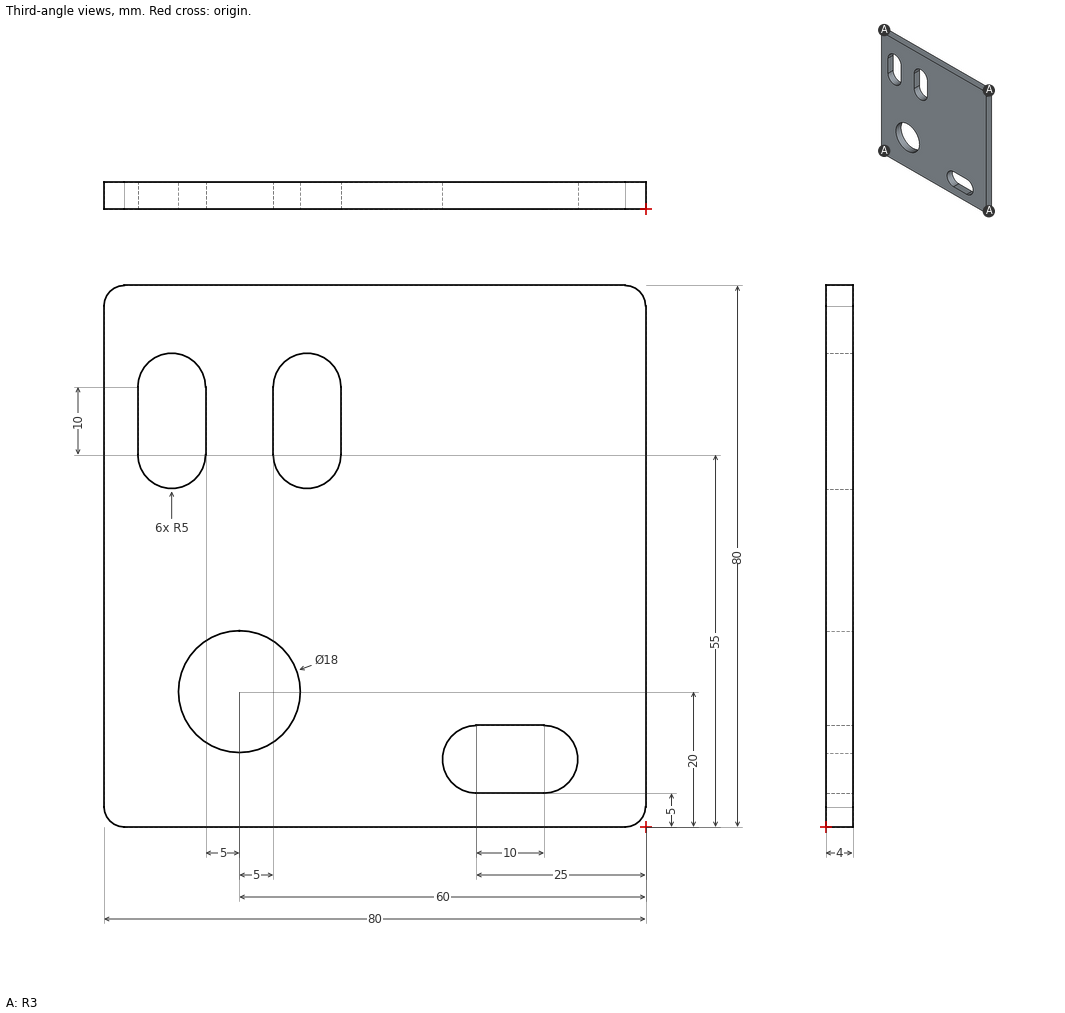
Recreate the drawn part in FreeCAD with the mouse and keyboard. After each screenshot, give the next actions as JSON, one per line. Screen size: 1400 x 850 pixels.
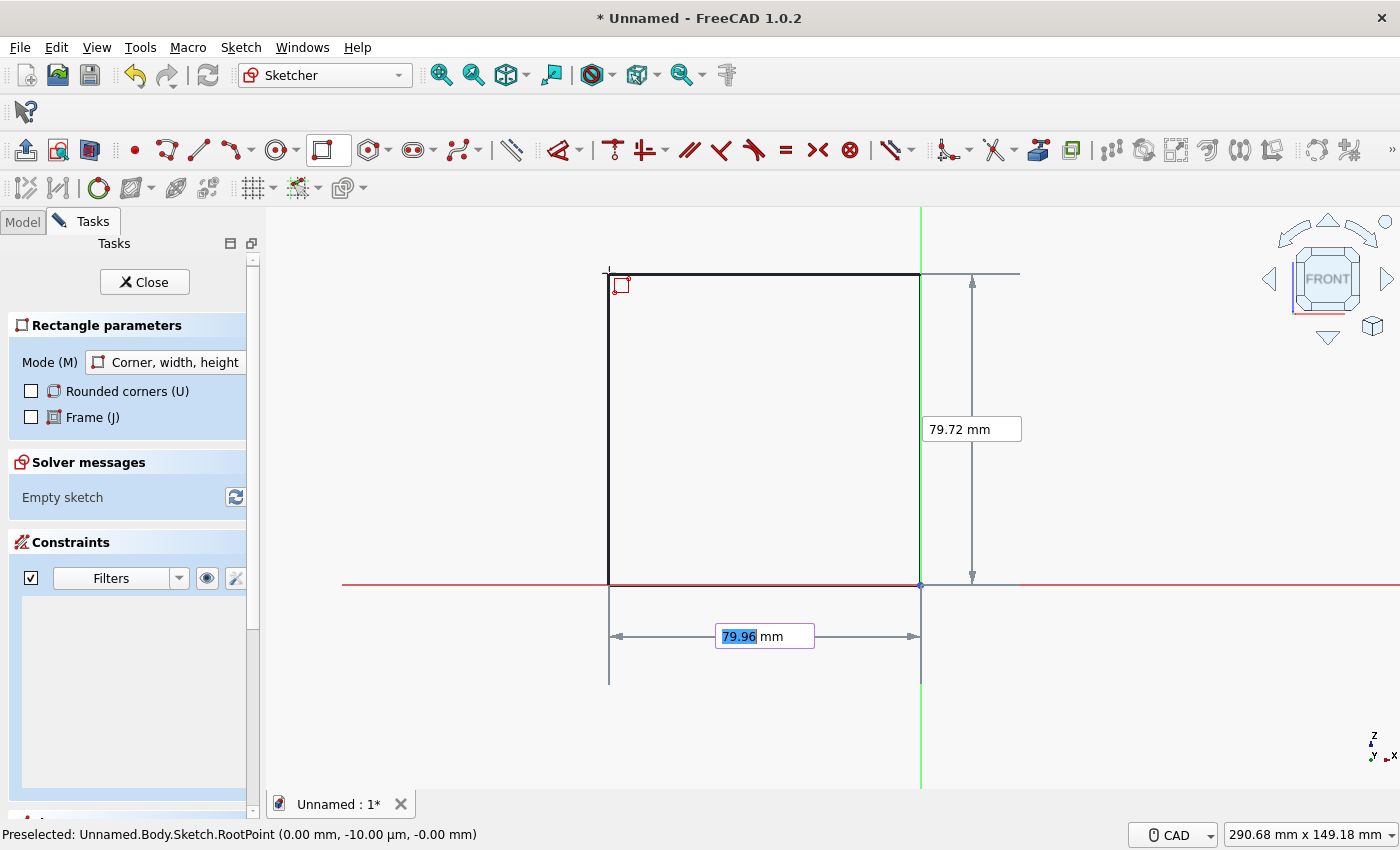
{"action": "type", "text": "80"}
{"action": "key", "text": "Tab"}
{"action": "type", "text": "80"}
{"action": "key", "text": "Return"}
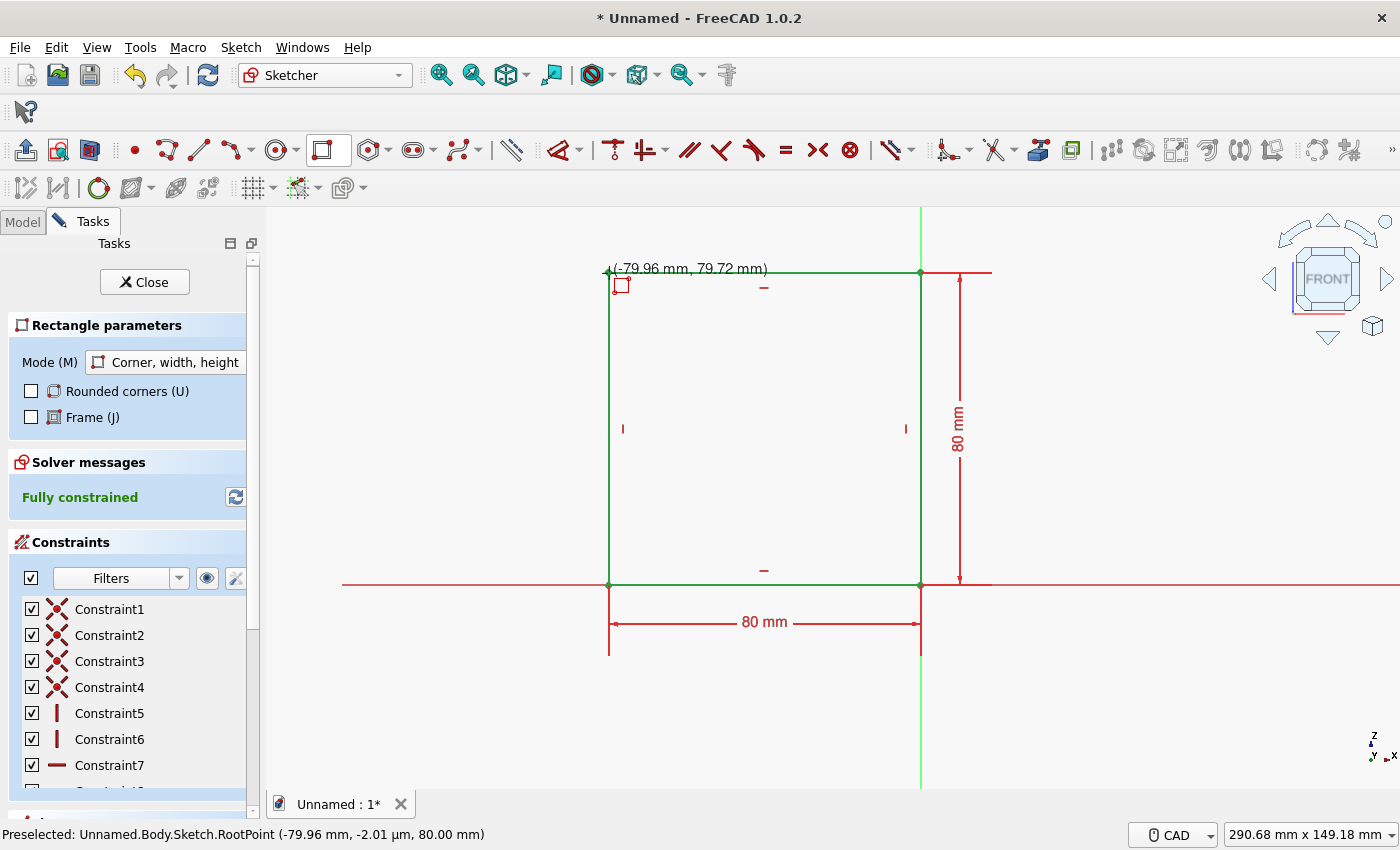
{"action": "left_click", "coordinate": [414, 150]}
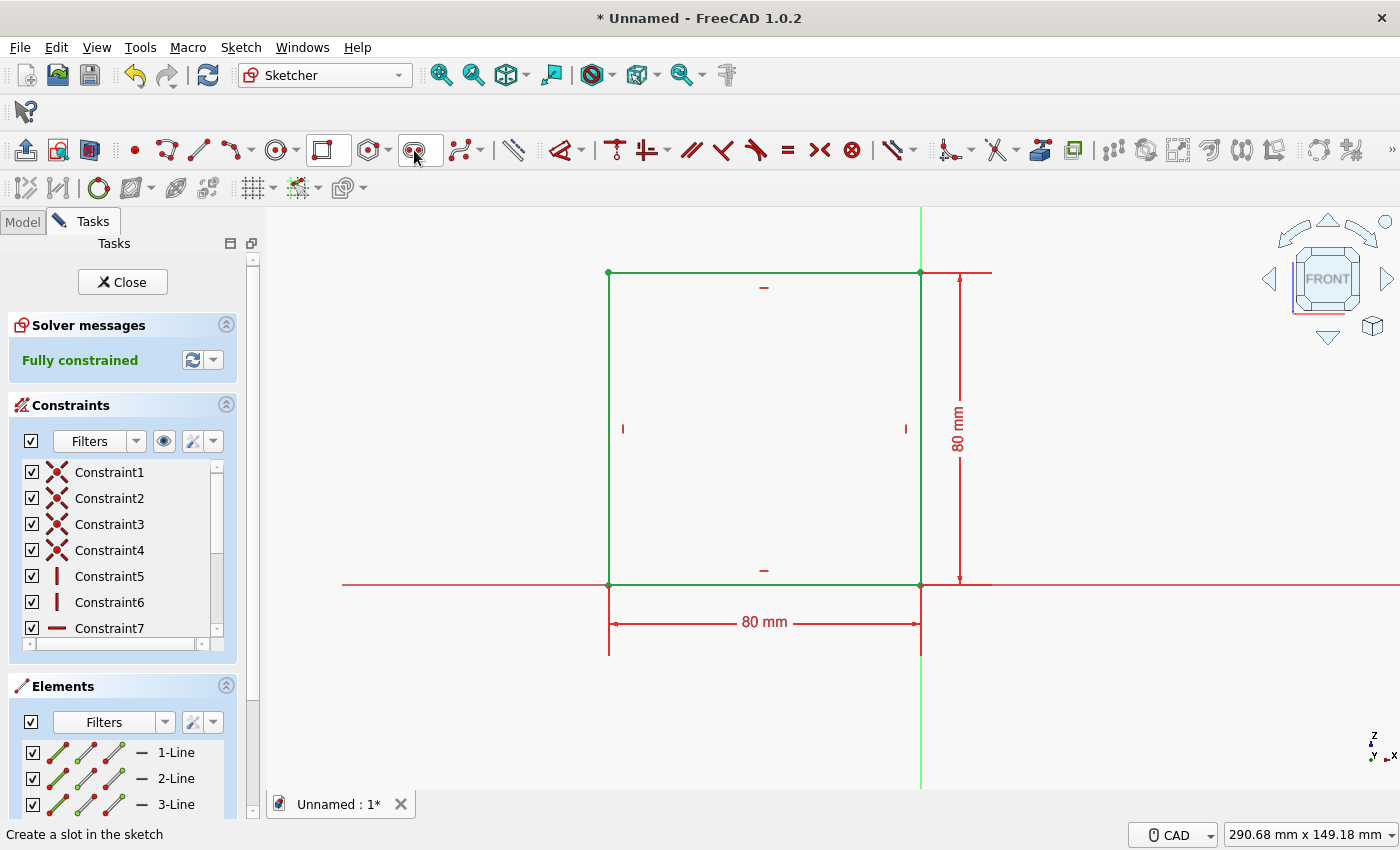
{"action": "left_click", "coordinate": [648, 370]}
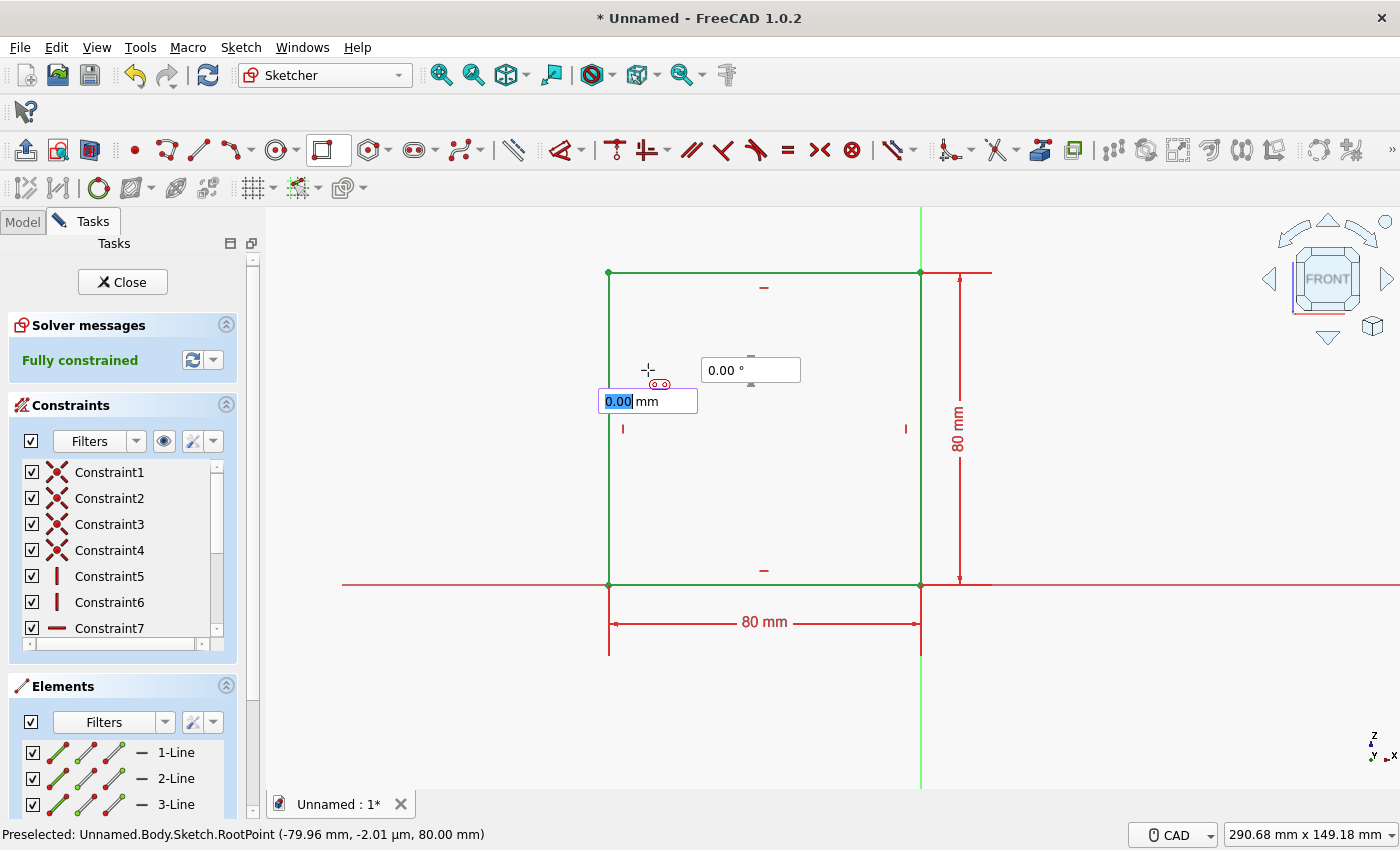
{"action": "left_click", "coordinate": [648, 331]}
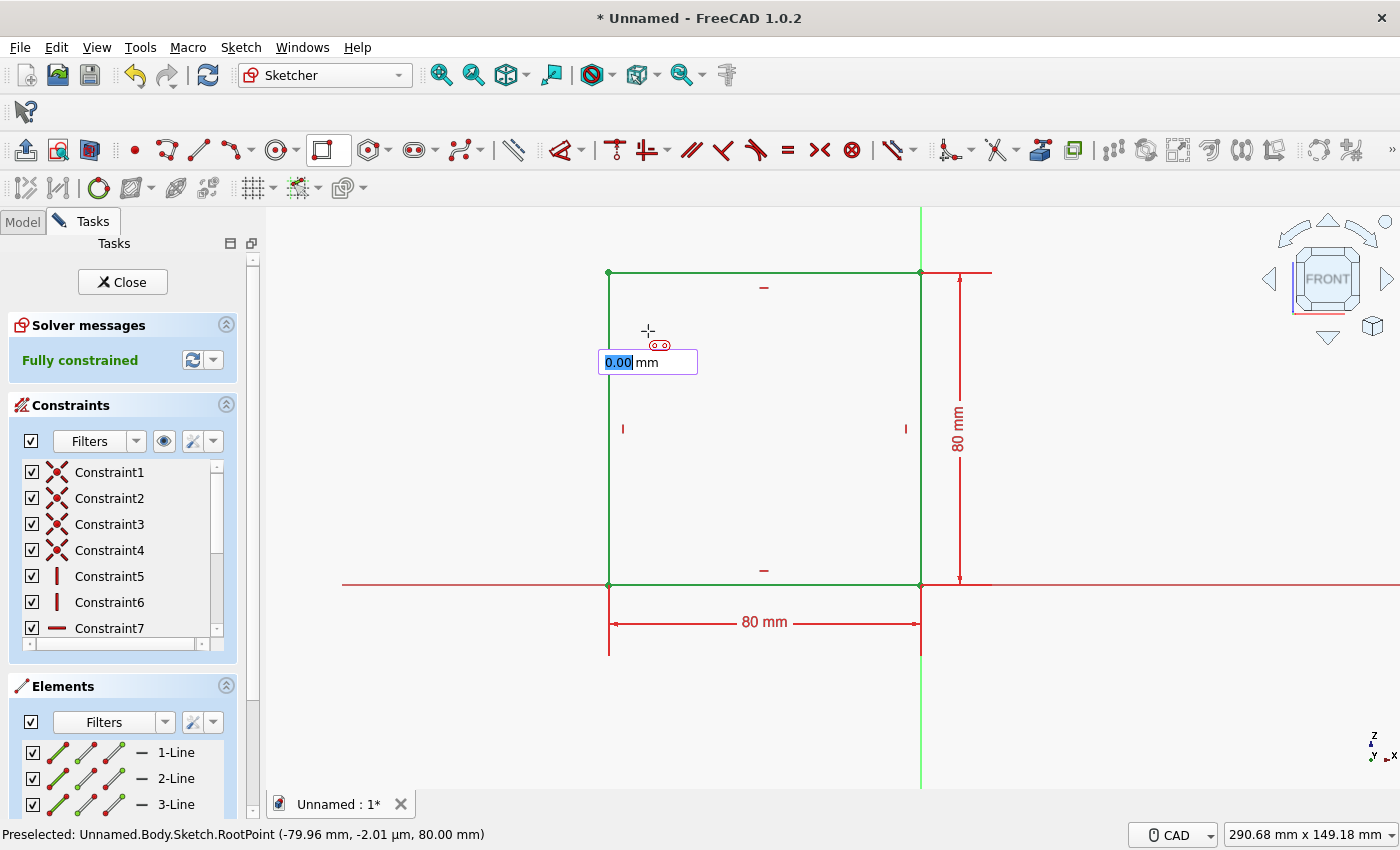
{"action": "left_click", "coordinate": [667, 351]}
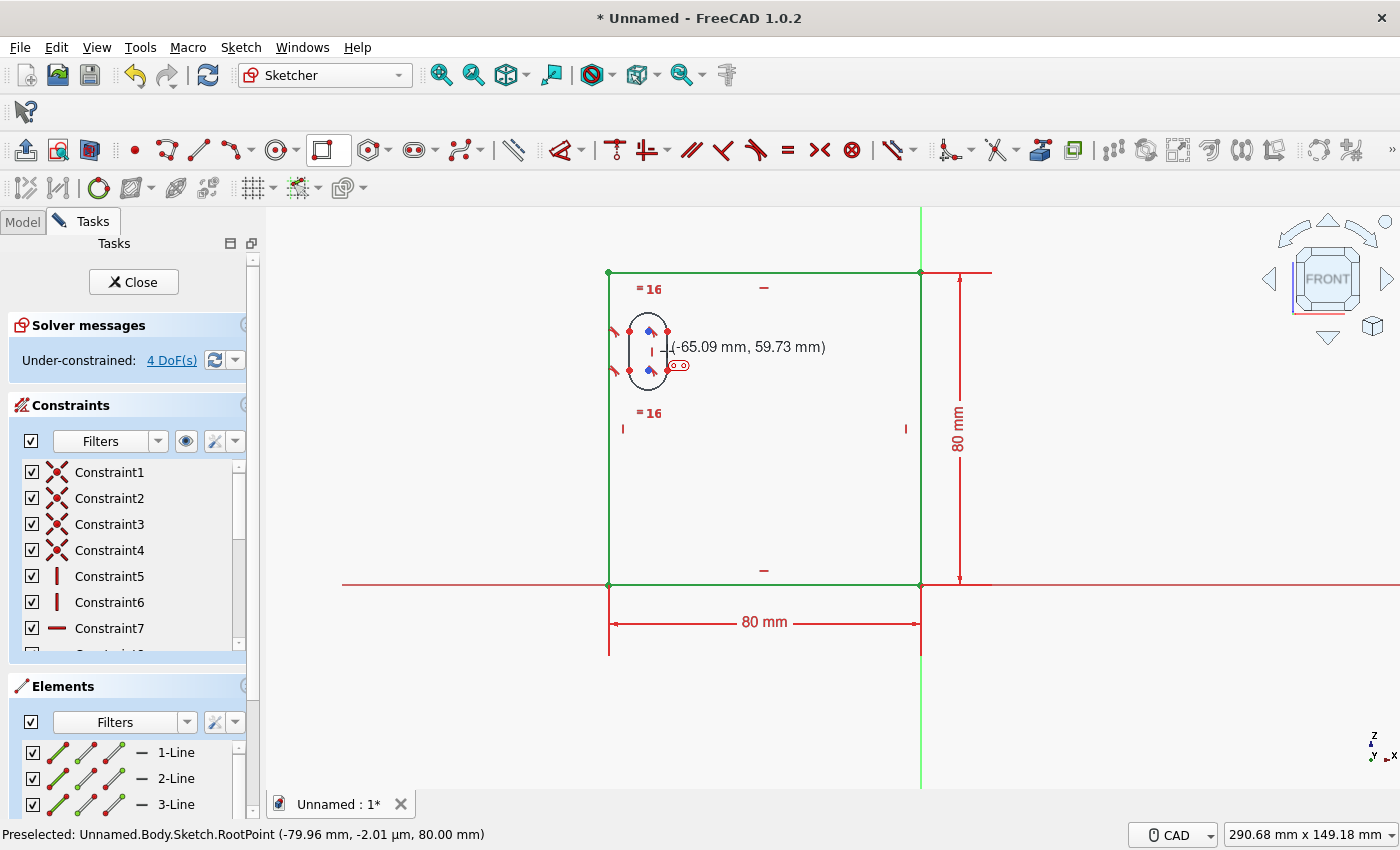
{"action": "left_click", "coordinate": [726, 370]}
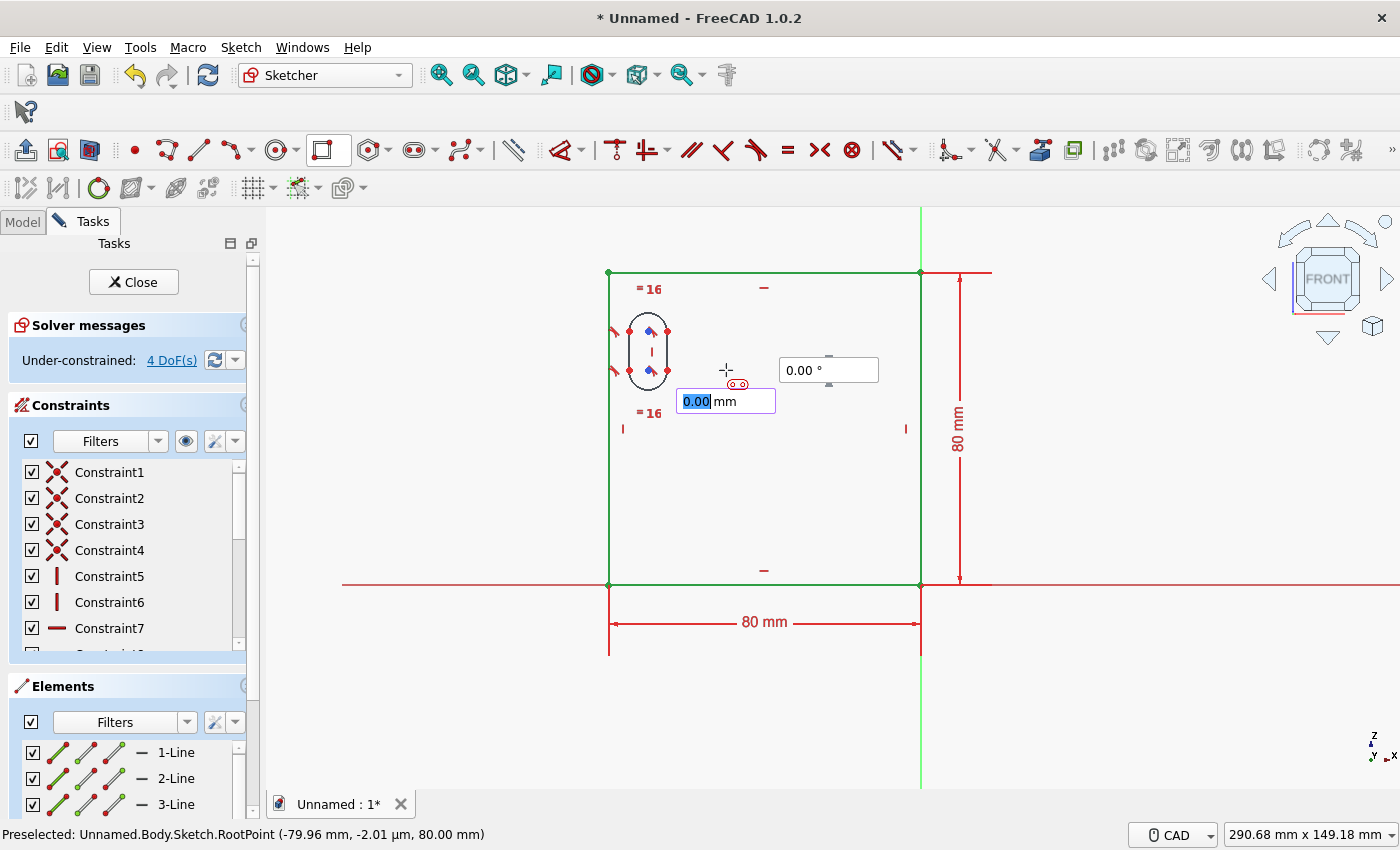
{"action": "left_click", "coordinate": [726, 331]}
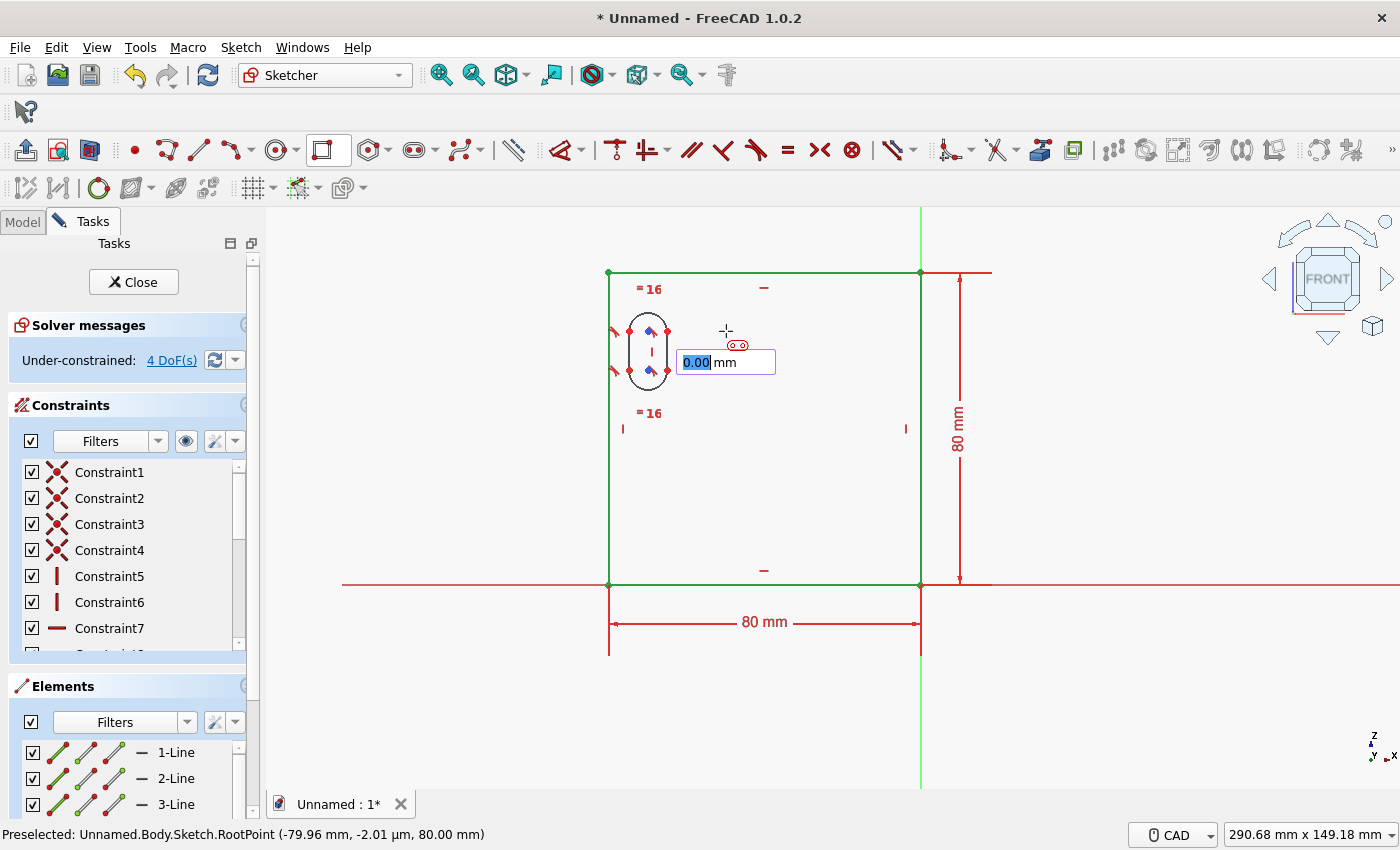
{"action": "left_click", "coordinate": [745, 351]}